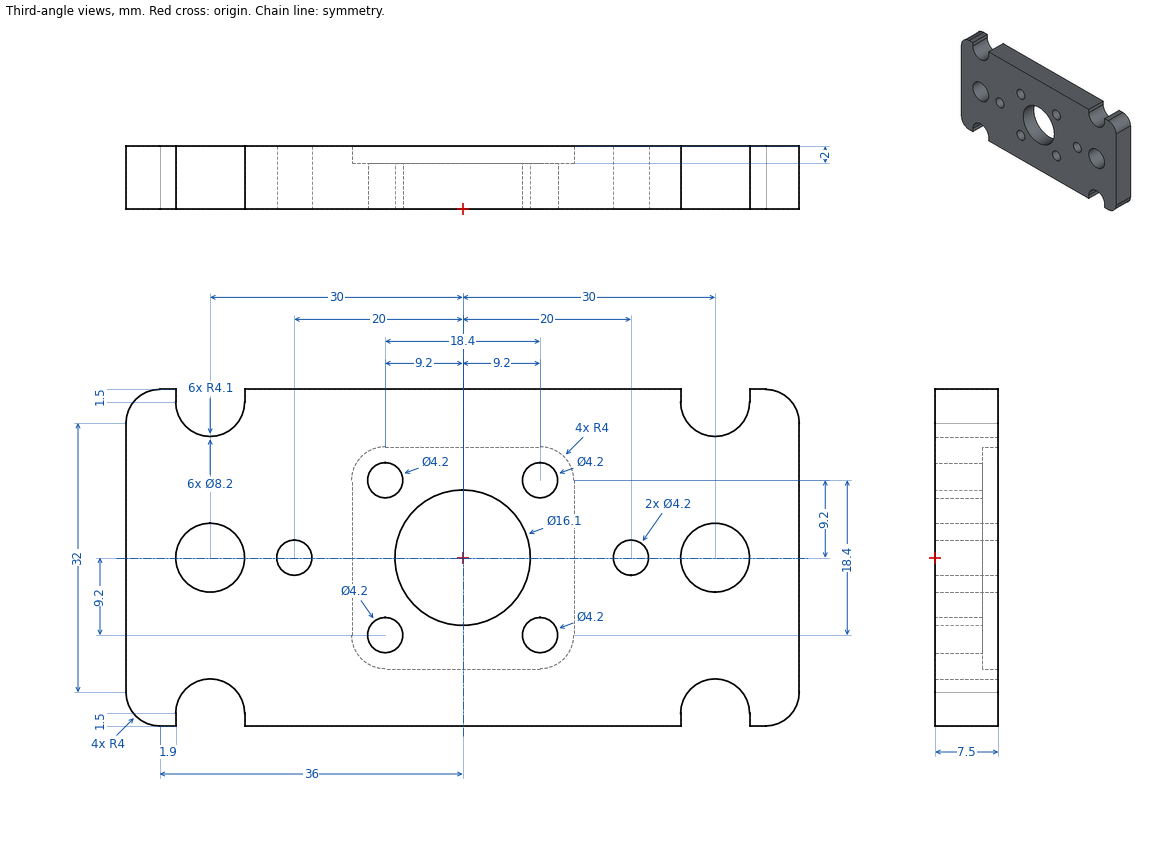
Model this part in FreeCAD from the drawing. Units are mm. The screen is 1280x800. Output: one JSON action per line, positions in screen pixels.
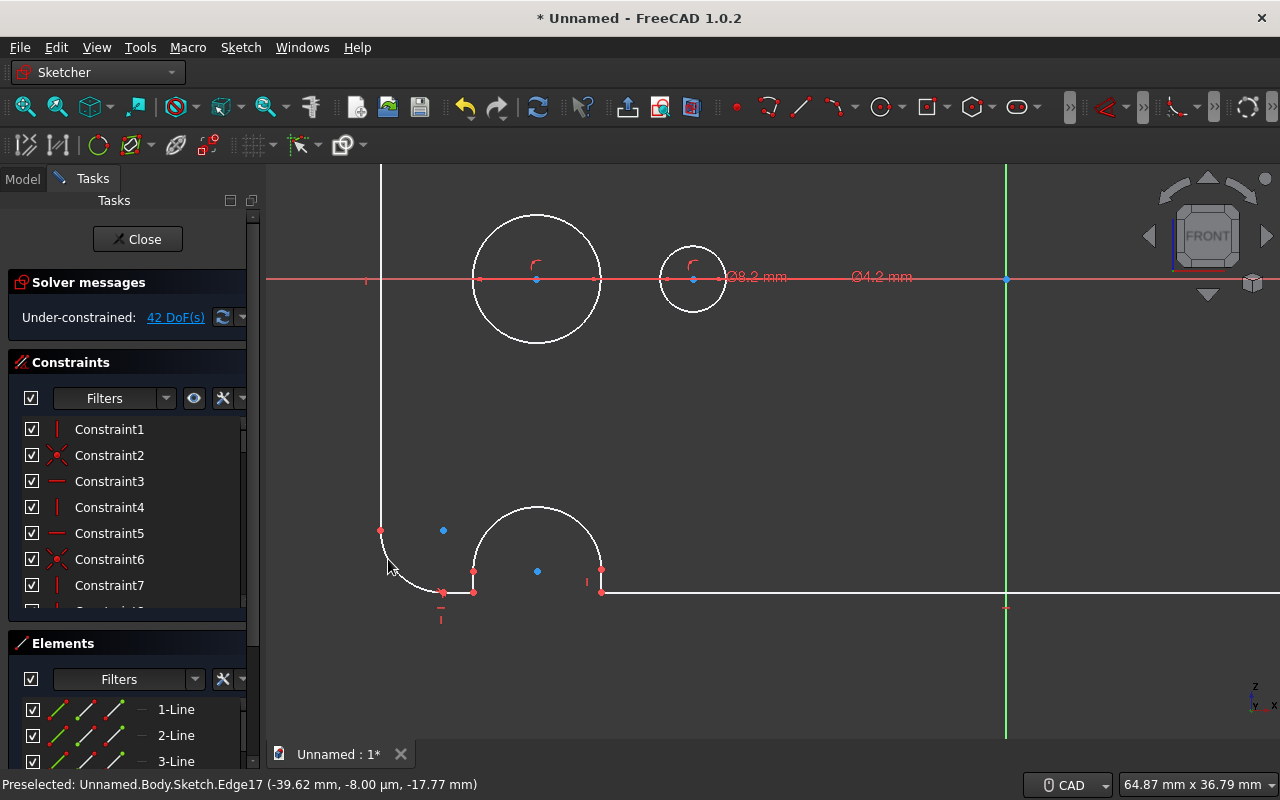
{"action": "left_click", "coordinate": [381, 380]}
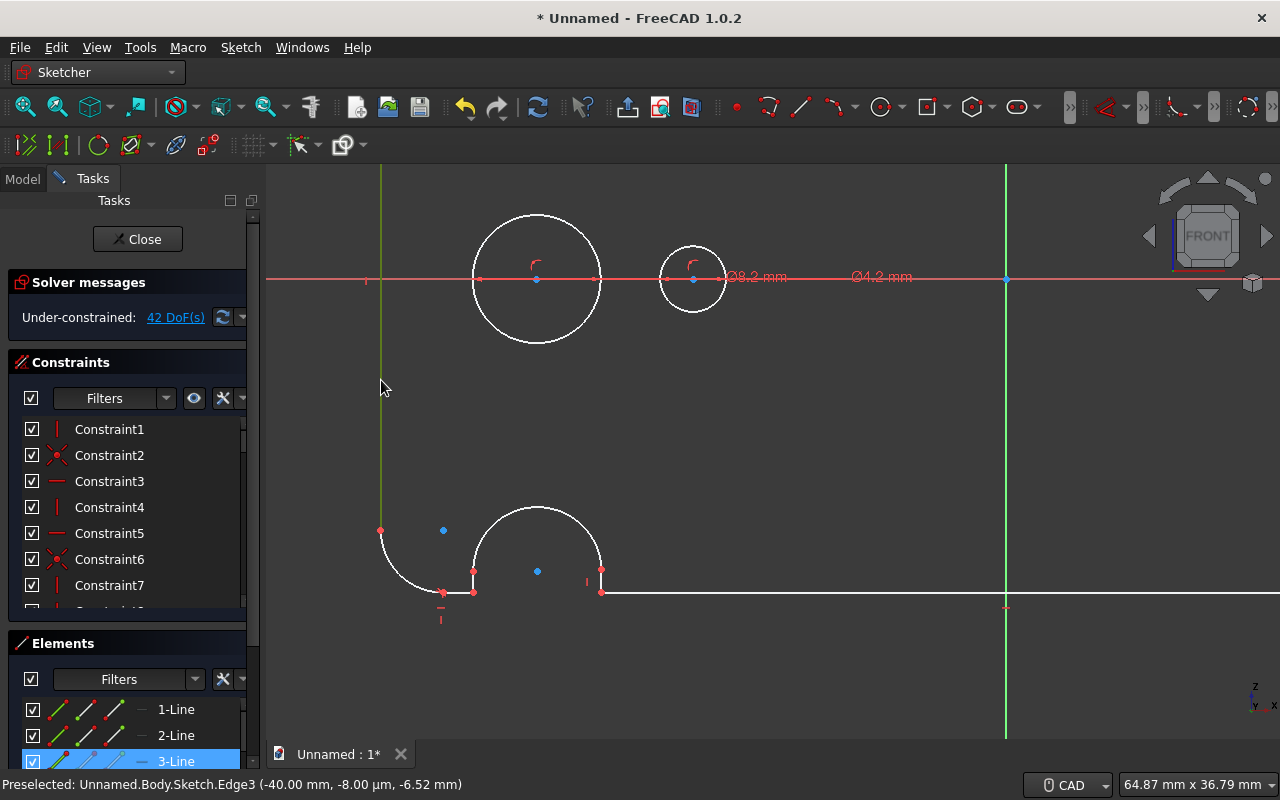
{"action": "left_click", "coordinate": [388, 559]}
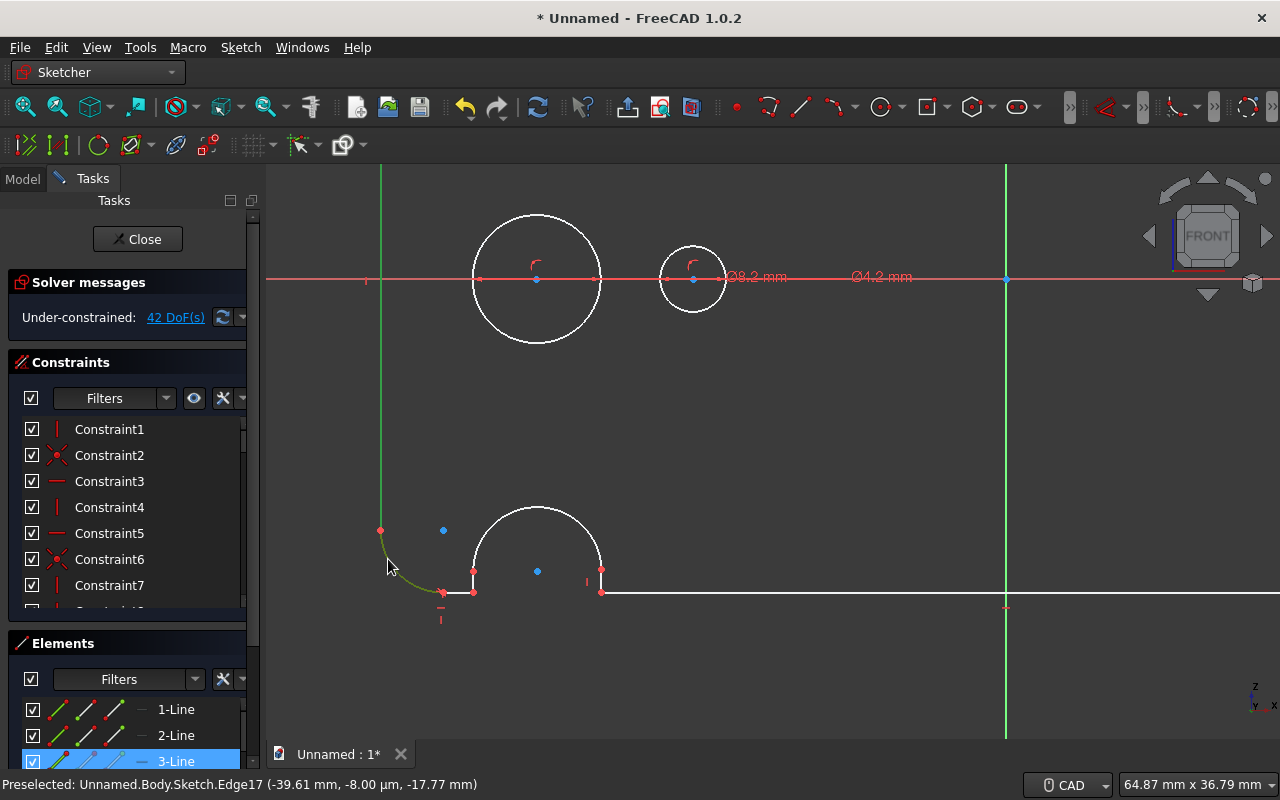
{"action": "key", "text": "t"}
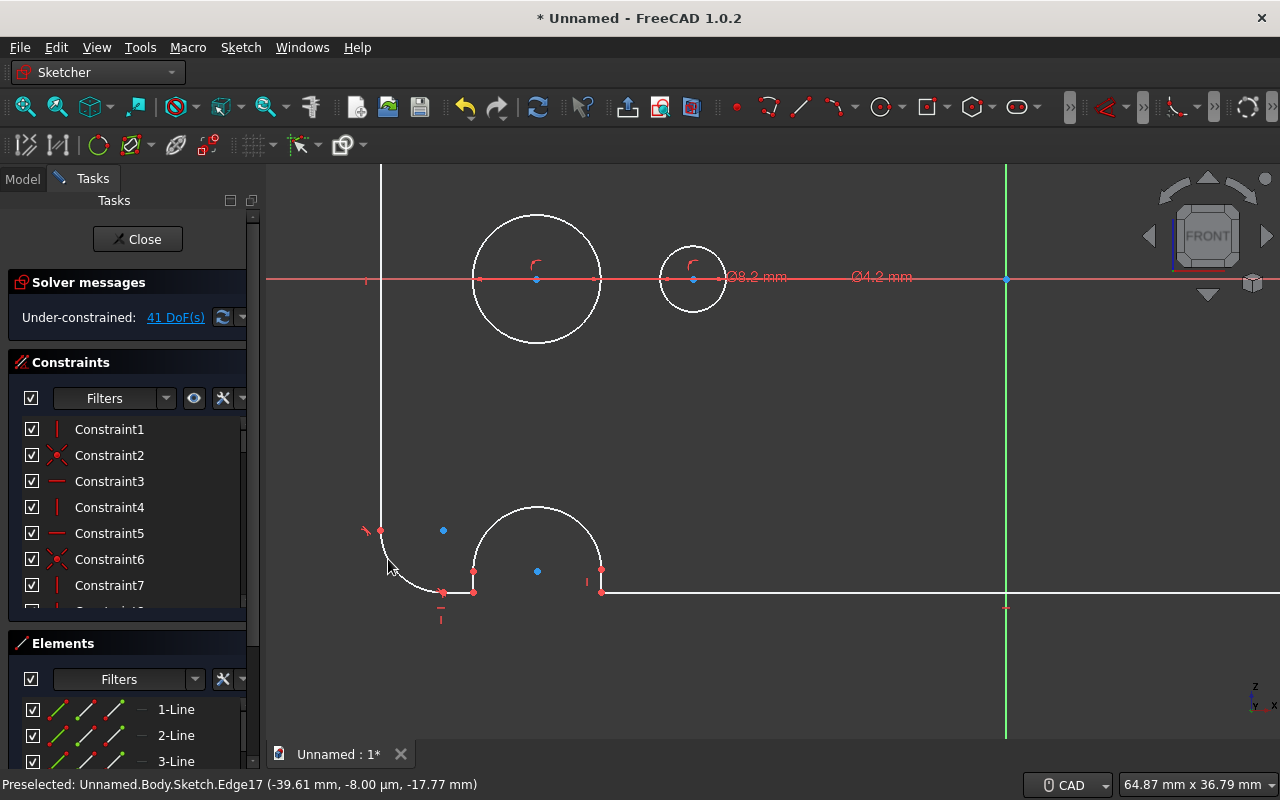
{"action": "left_click", "coordinate": [381, 380]}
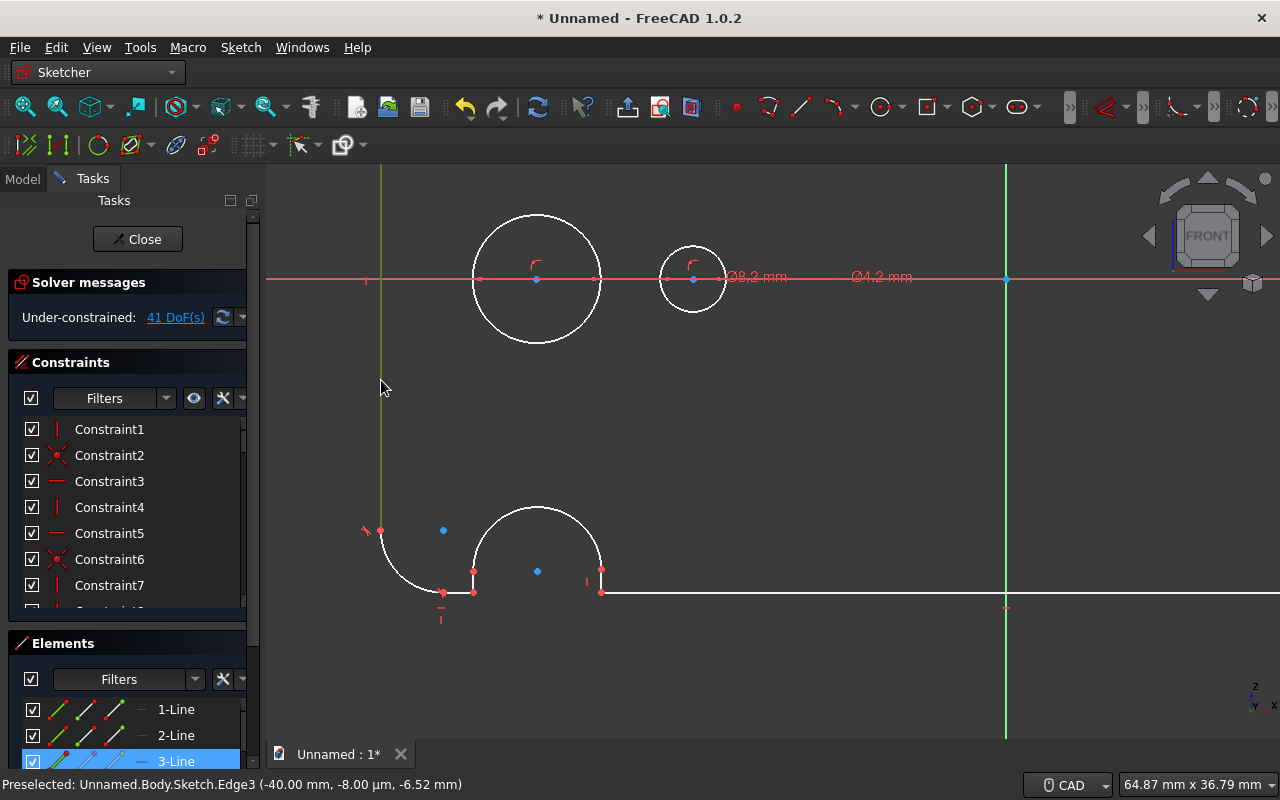
{"action": "scroll", "coordinate": [458, 592], "scroll_direction": "down", "scroll_amount": 4}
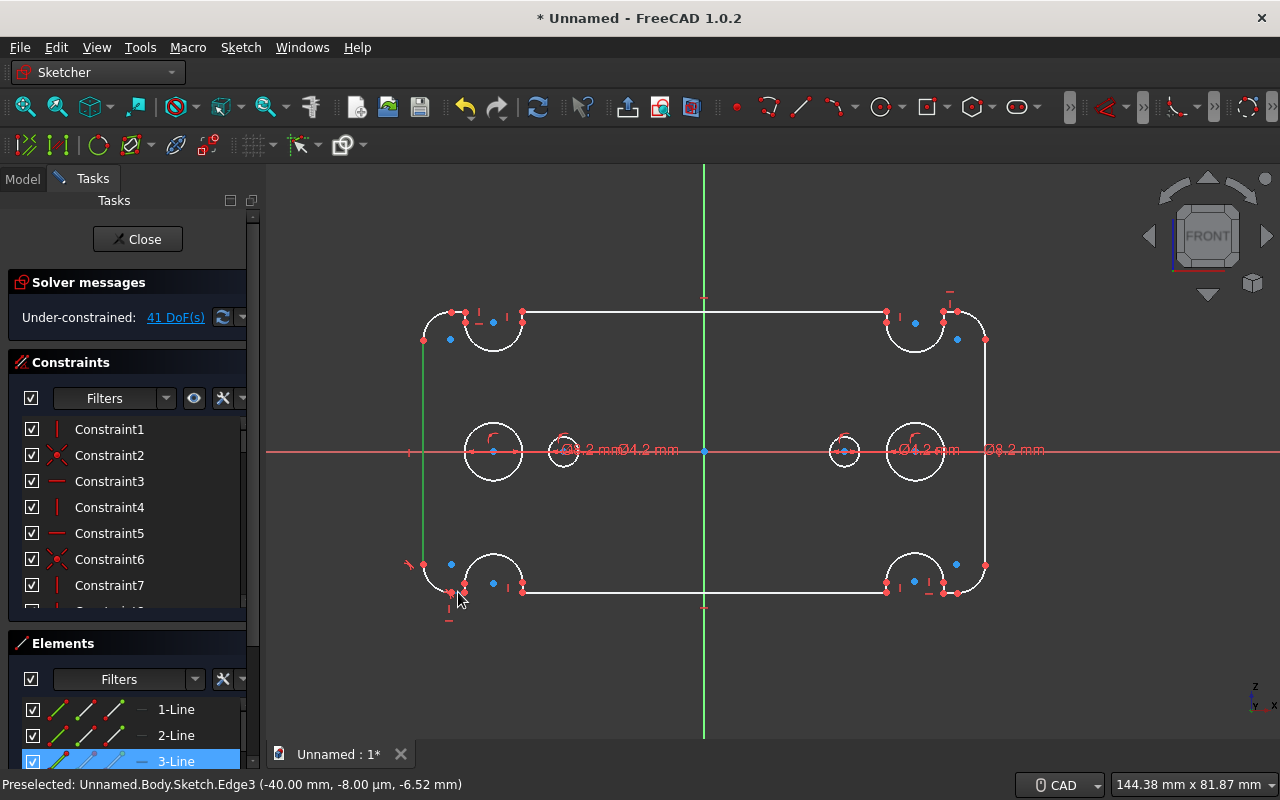
{"action": "left_click", "coordinate": [438, 315]}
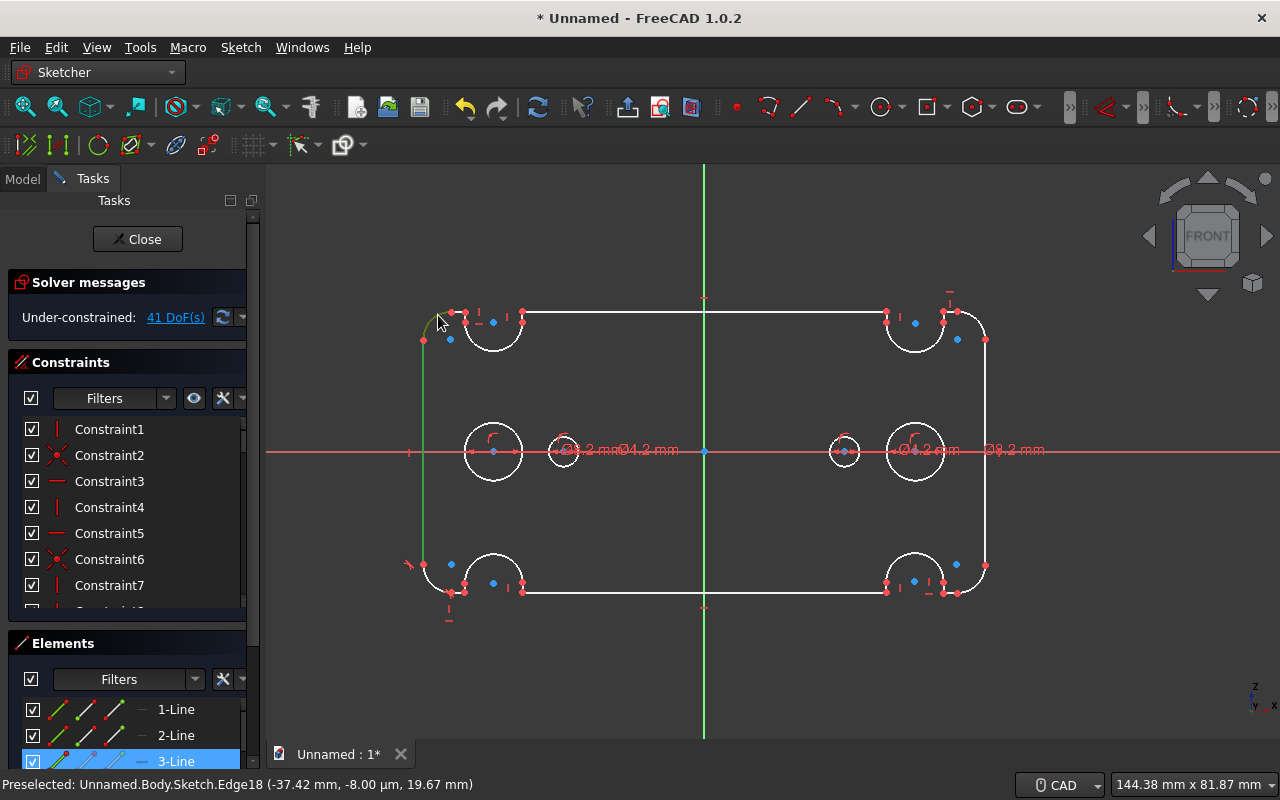
{"action": "key", "text": "t"}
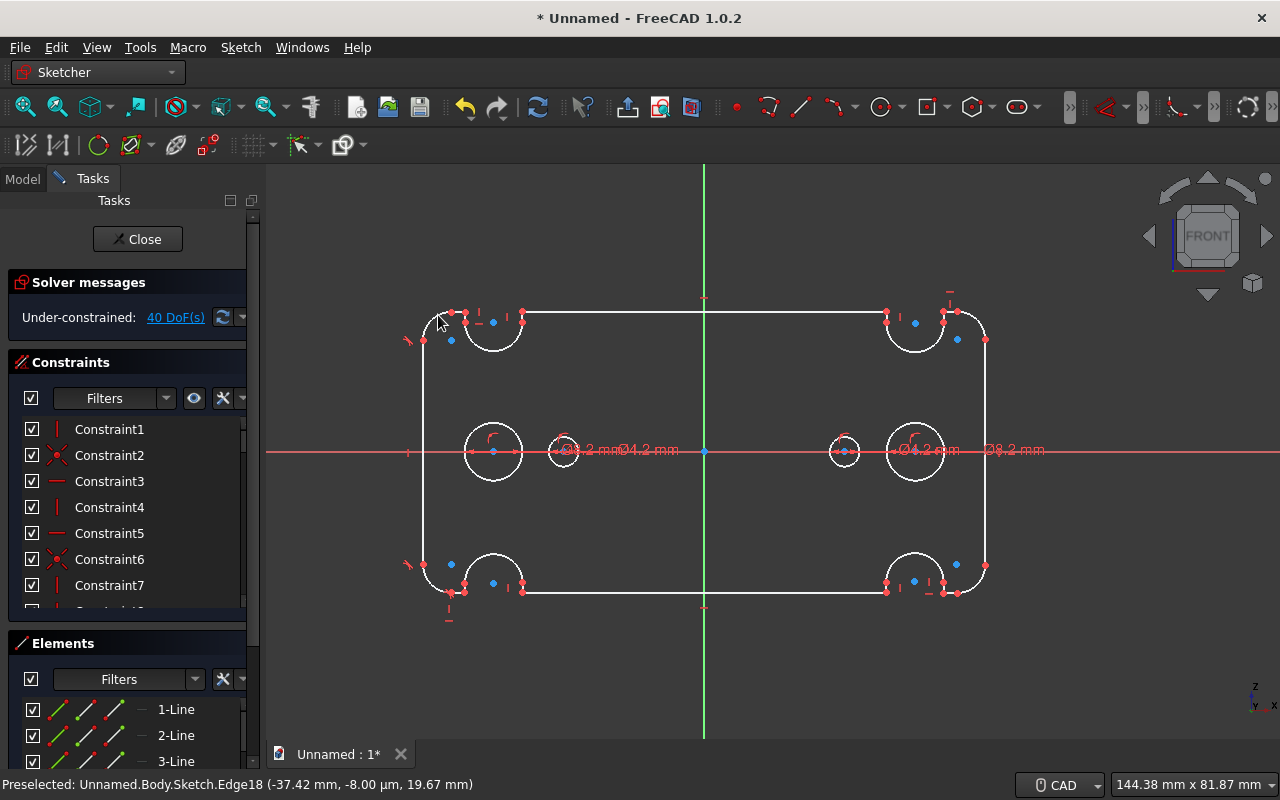
{"action": "scroll", "coordinate": [458, 312], "scroll_direction": "up", "scroll_amount": 4}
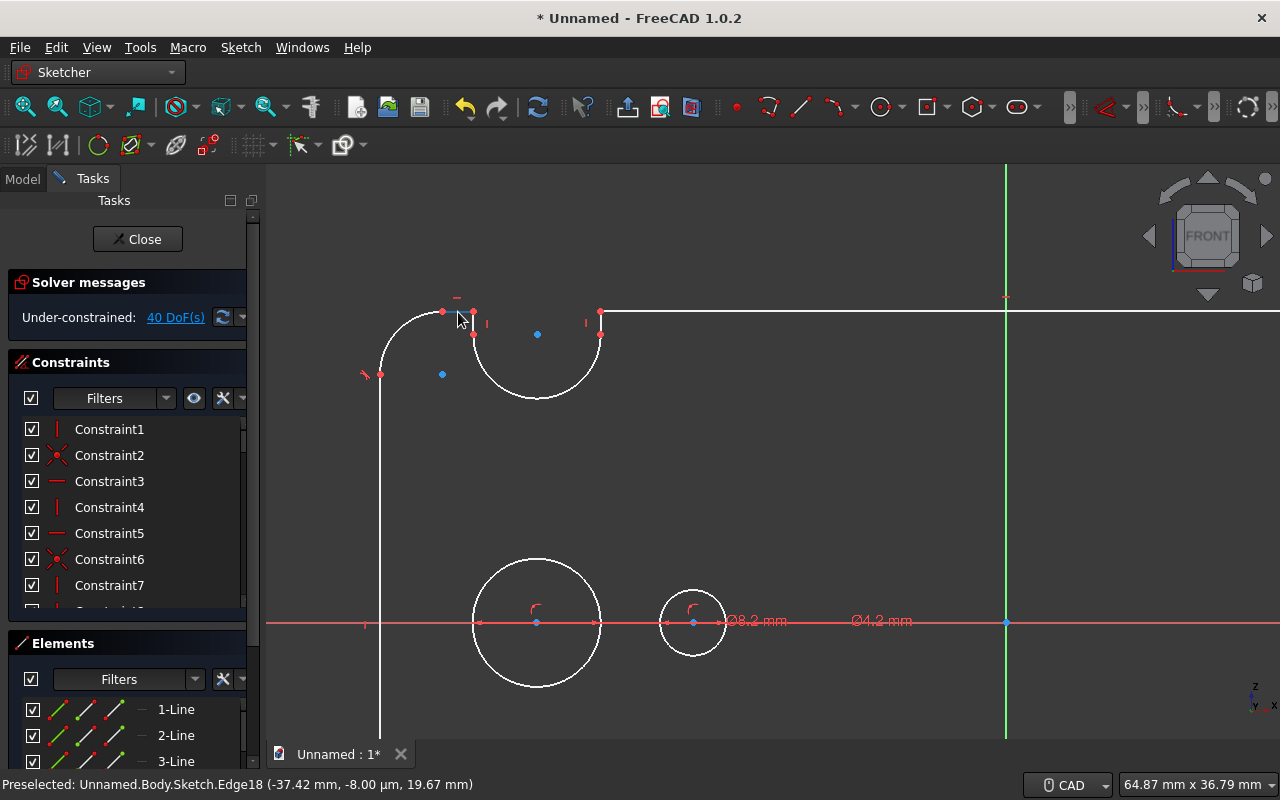
{"action": "left_click", "coordinate": [458, 312]}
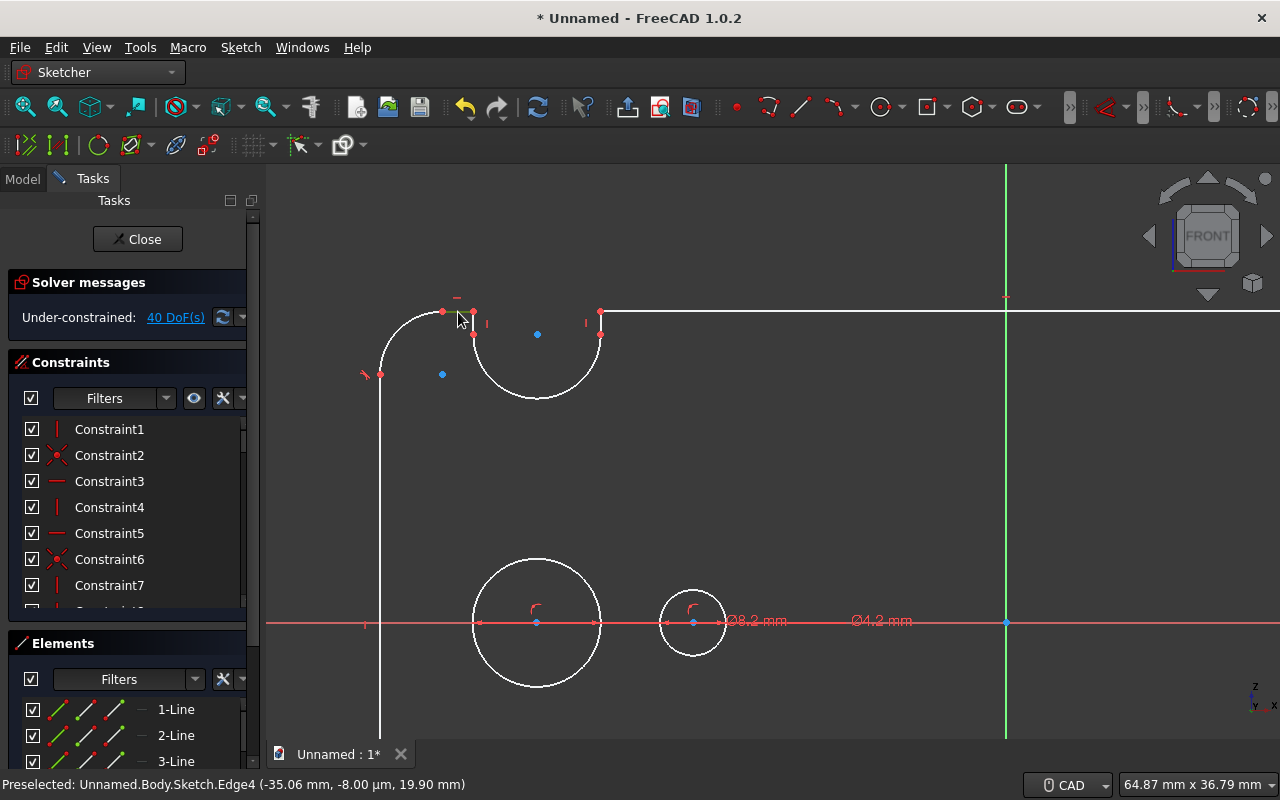
{"action": "left_click", "coordinate": [414, 319]}